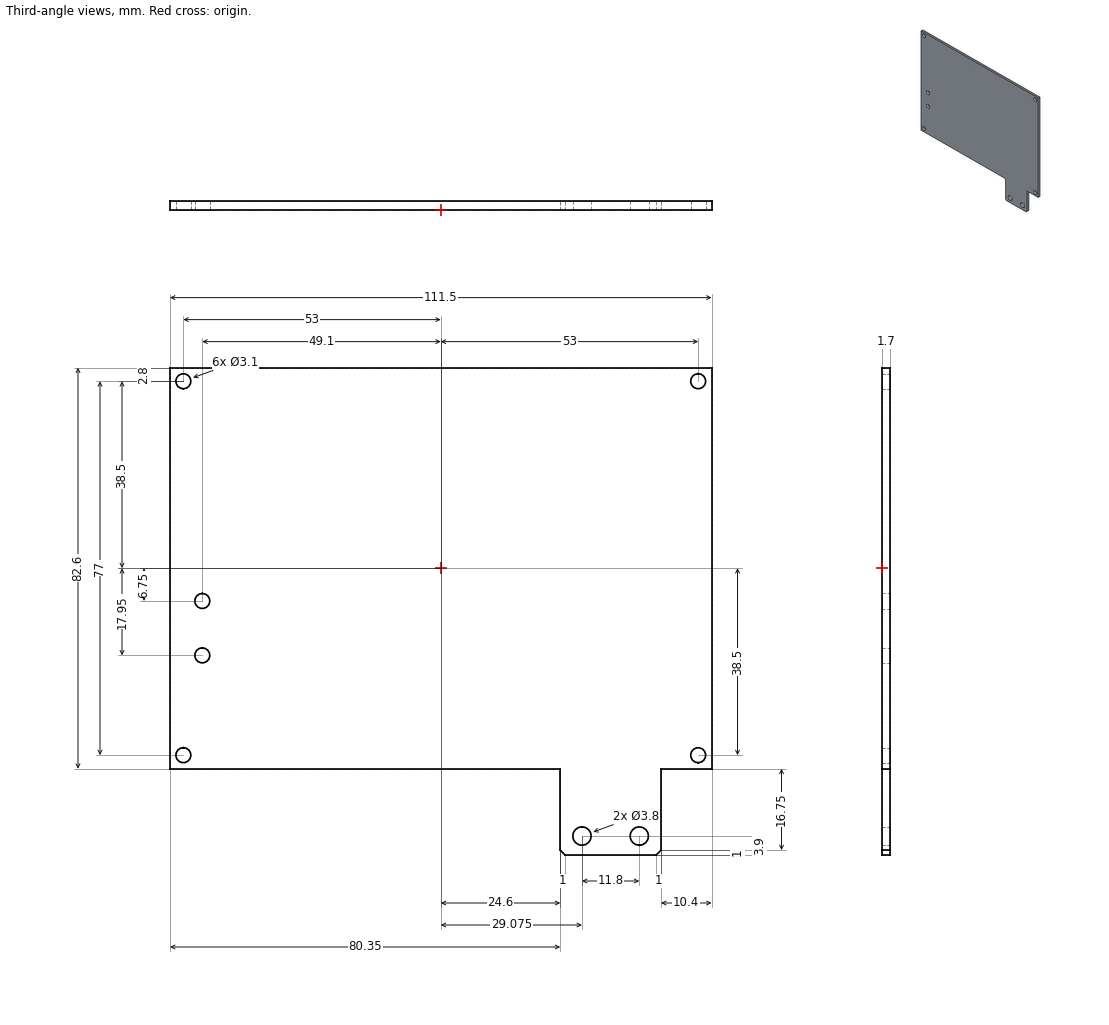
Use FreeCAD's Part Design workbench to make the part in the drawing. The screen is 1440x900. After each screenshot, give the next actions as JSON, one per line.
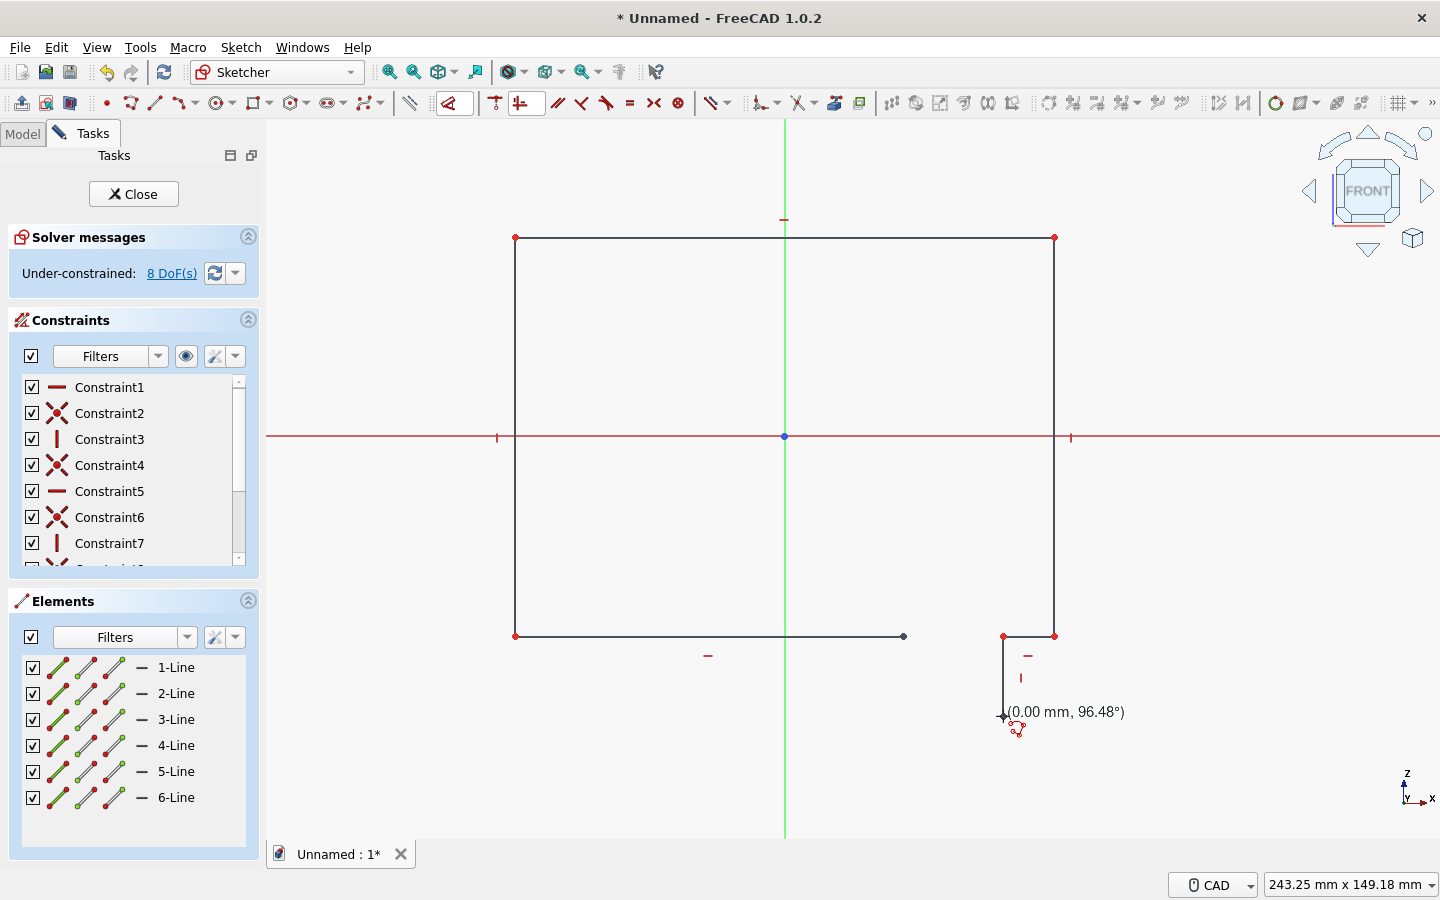
{"action": "scroll", "coordinate": [999, 721], "scroll_direction": "up", "scroll_amount": 5}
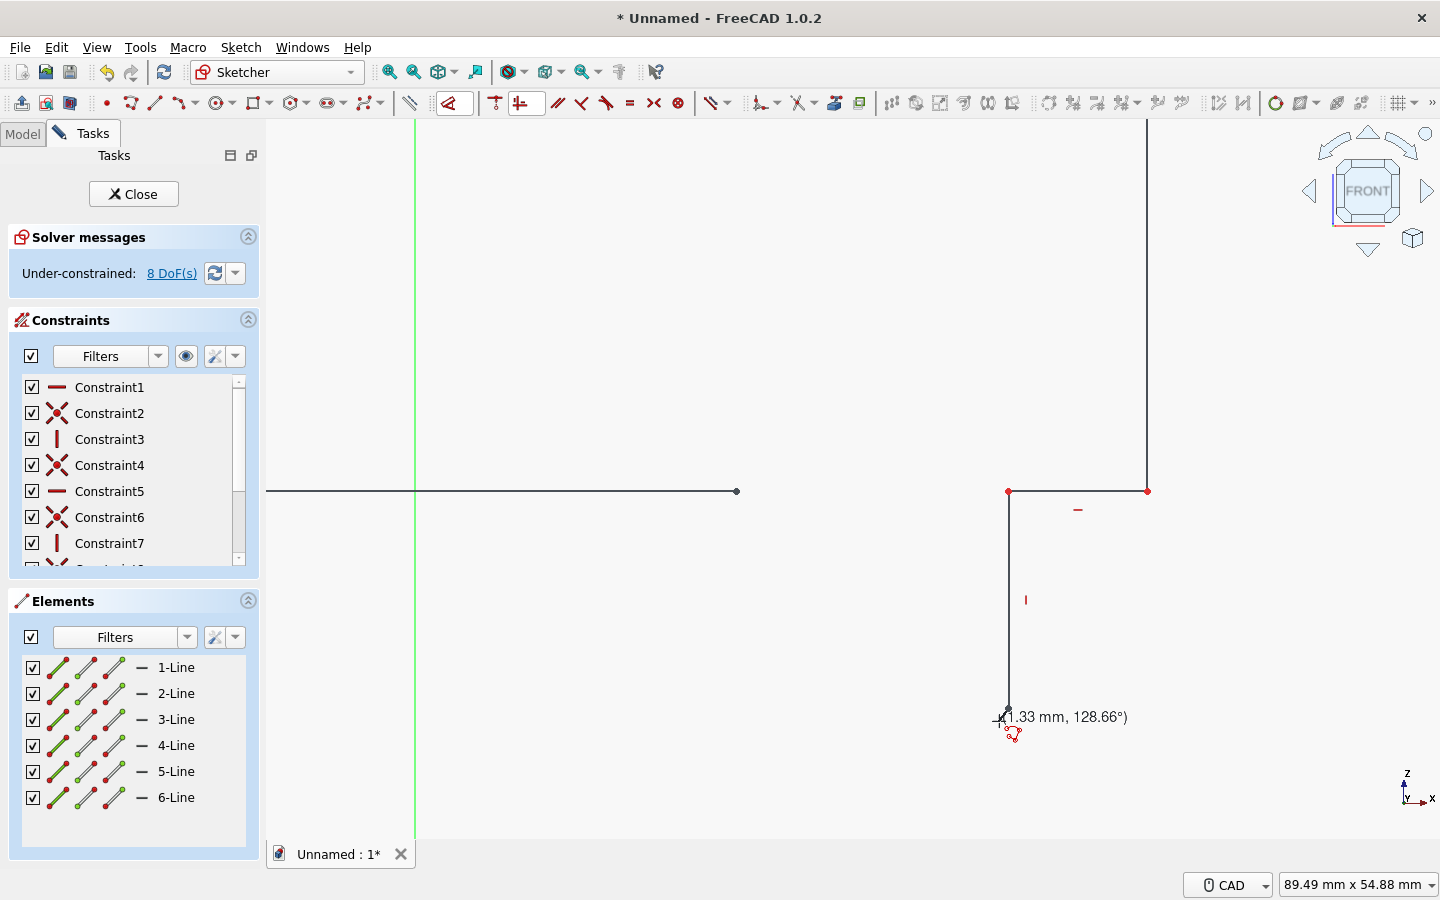
{"action": "left_click", "coordinate": [997, 720]}
{"action": "left_click", "coordinate": [751, 720]}
{"action": "left_click", "coordinate": [738, 707]}
{"action": "left_click", "coordinate": [737, 491]}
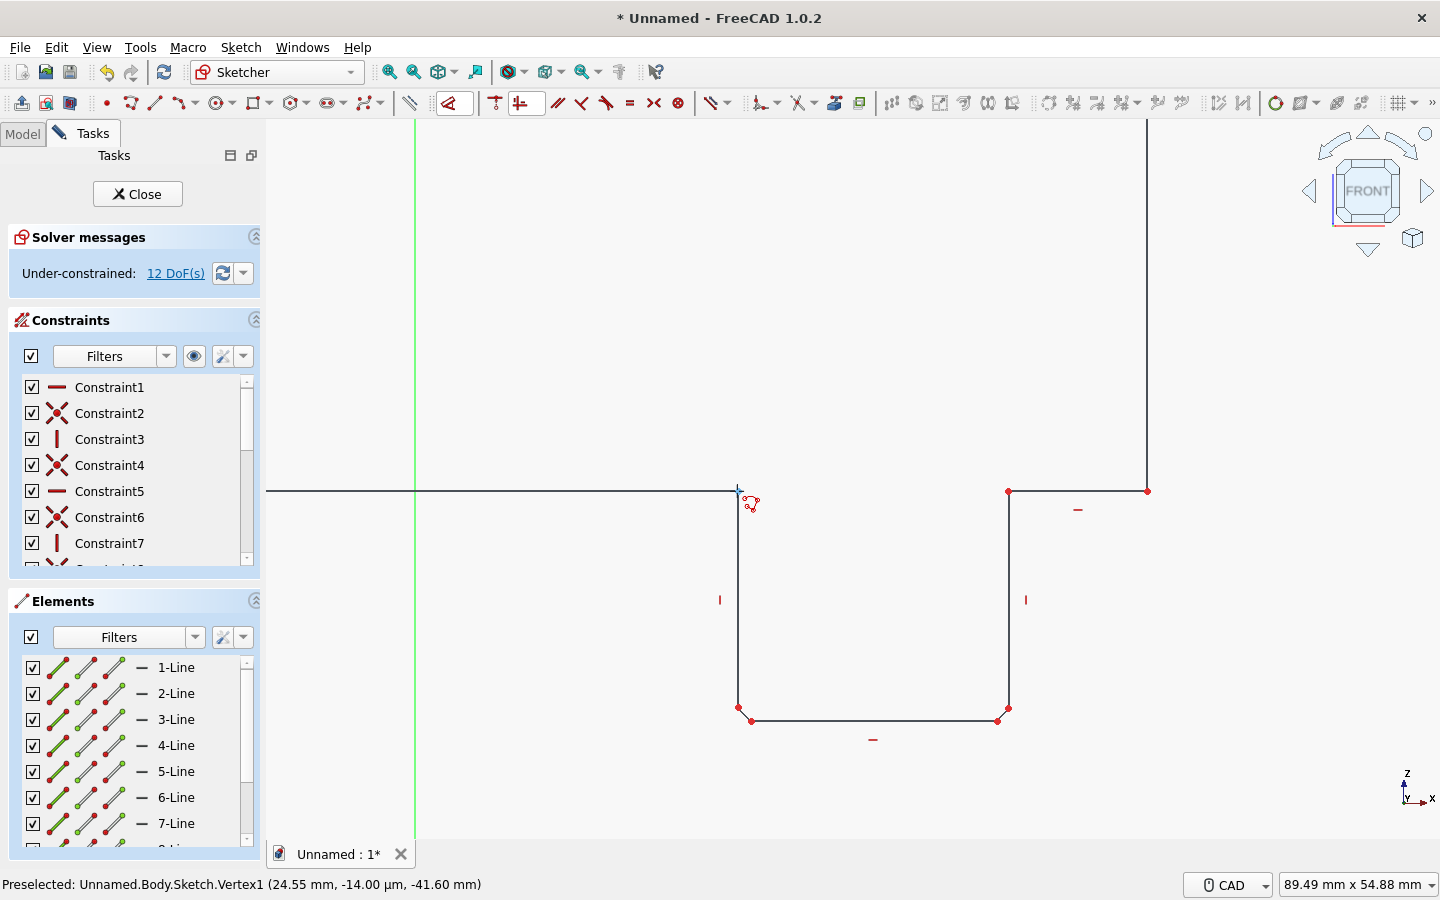
{"action": "left_click", "coordinate": [216, 104]}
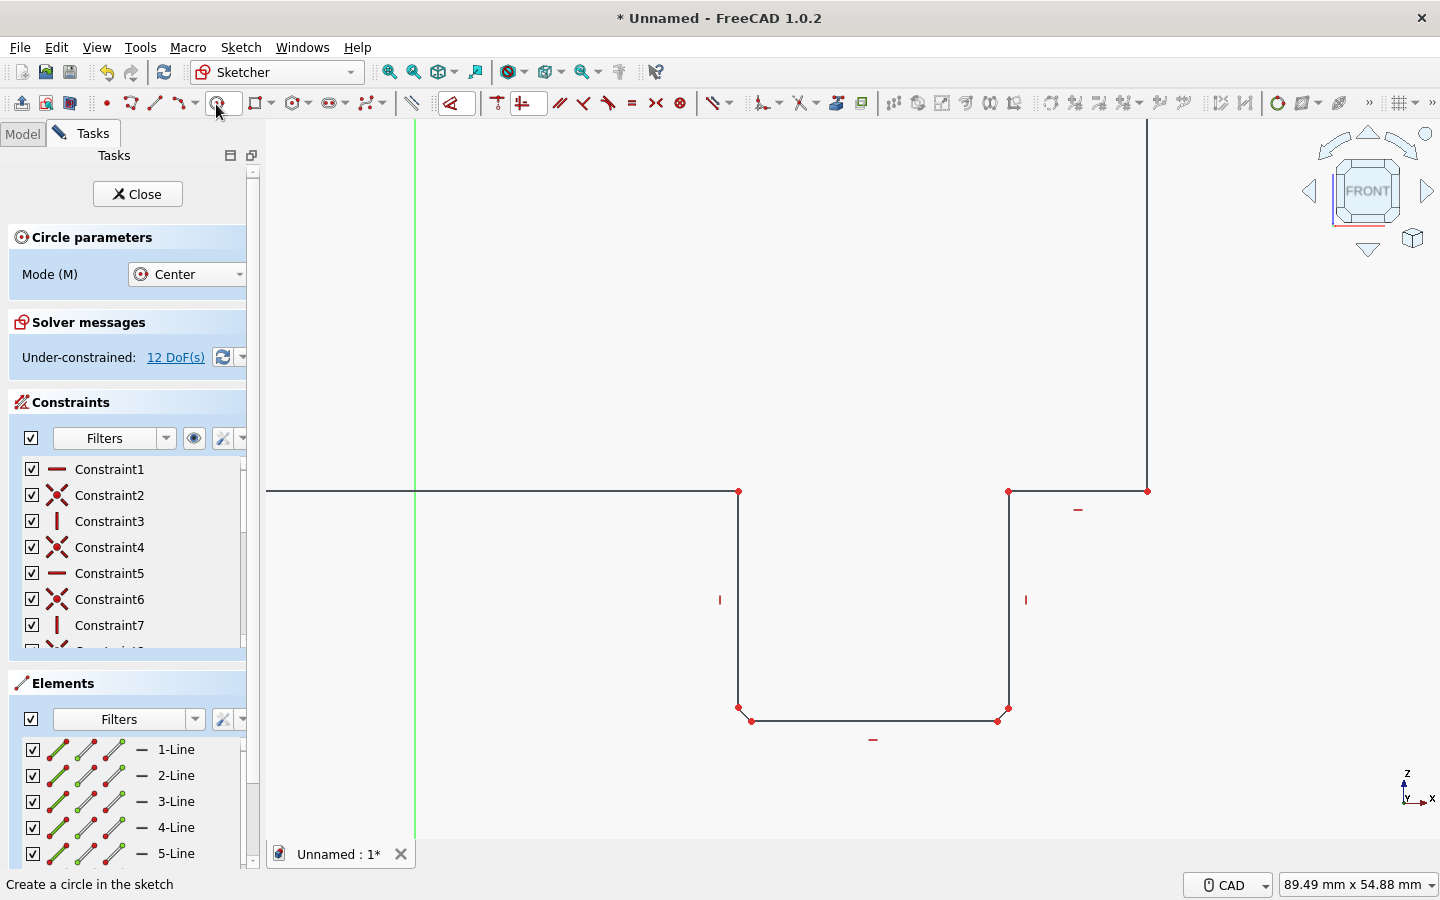
{"action": "scroll", "coordinate": [1000, 722], "scroll_direction": "down", "scroll_amount": 5}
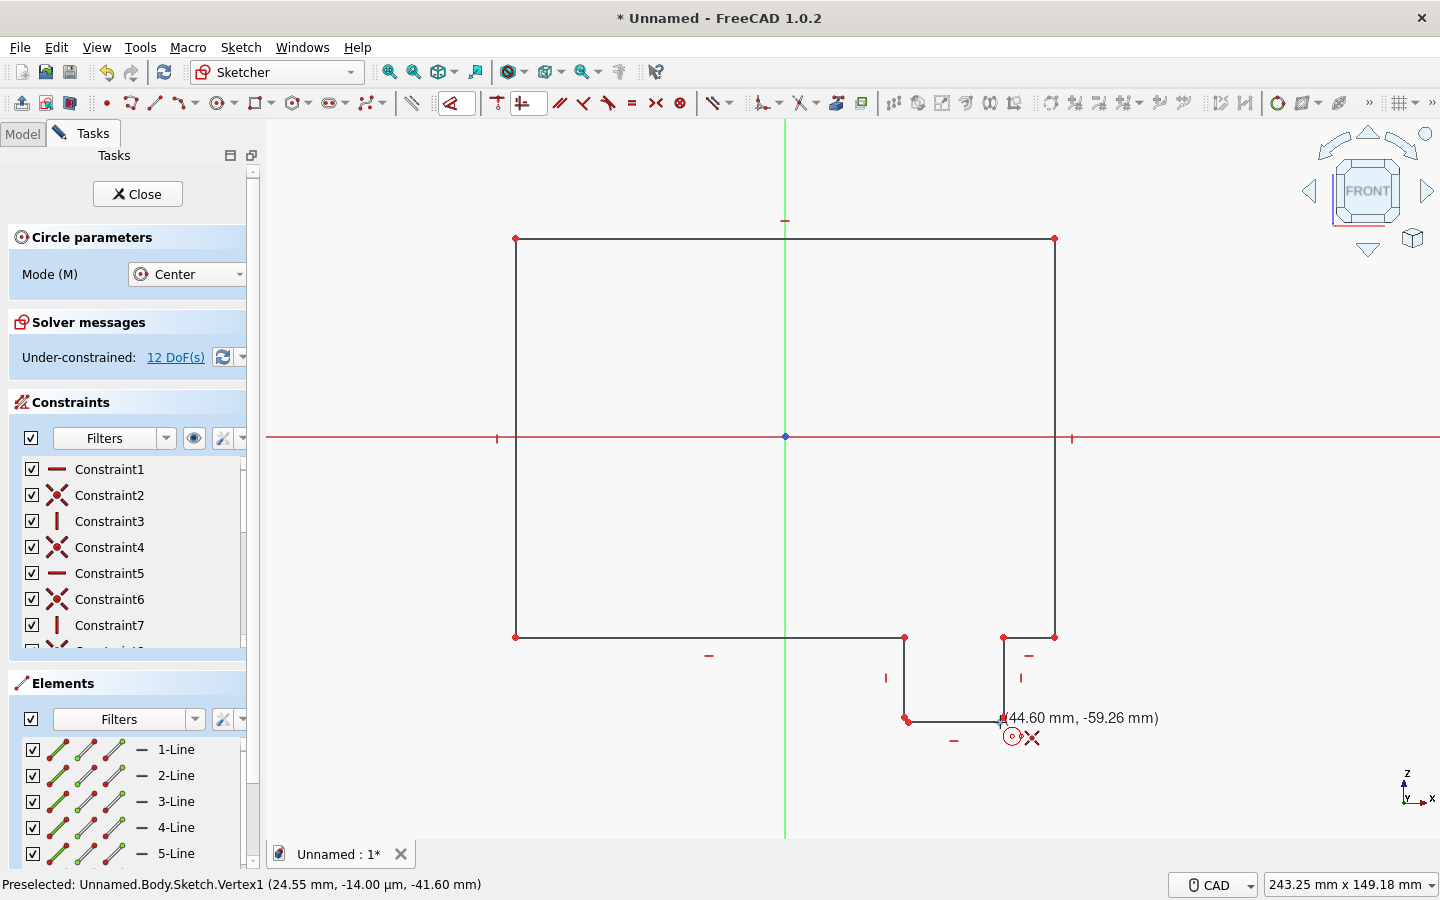
{"action": "scroll", "coordinate": [529, 251], "scroll_direction": "up", "scroll_amount": 6}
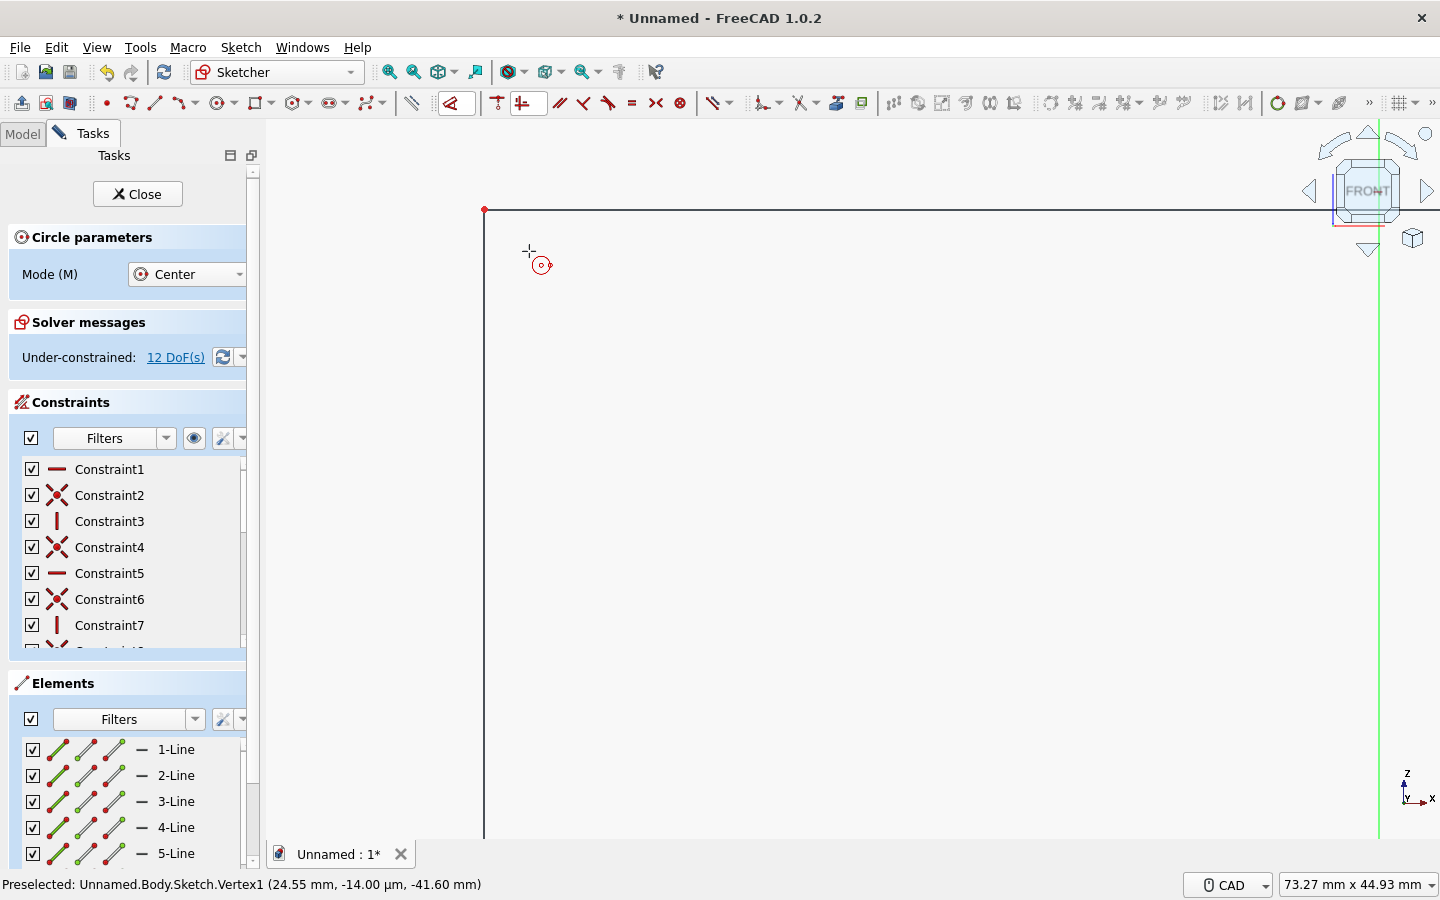
{"action": "left_click", "coordinate": [530, 251]}
{"action": "left_click", "coordinate": [547, 233]}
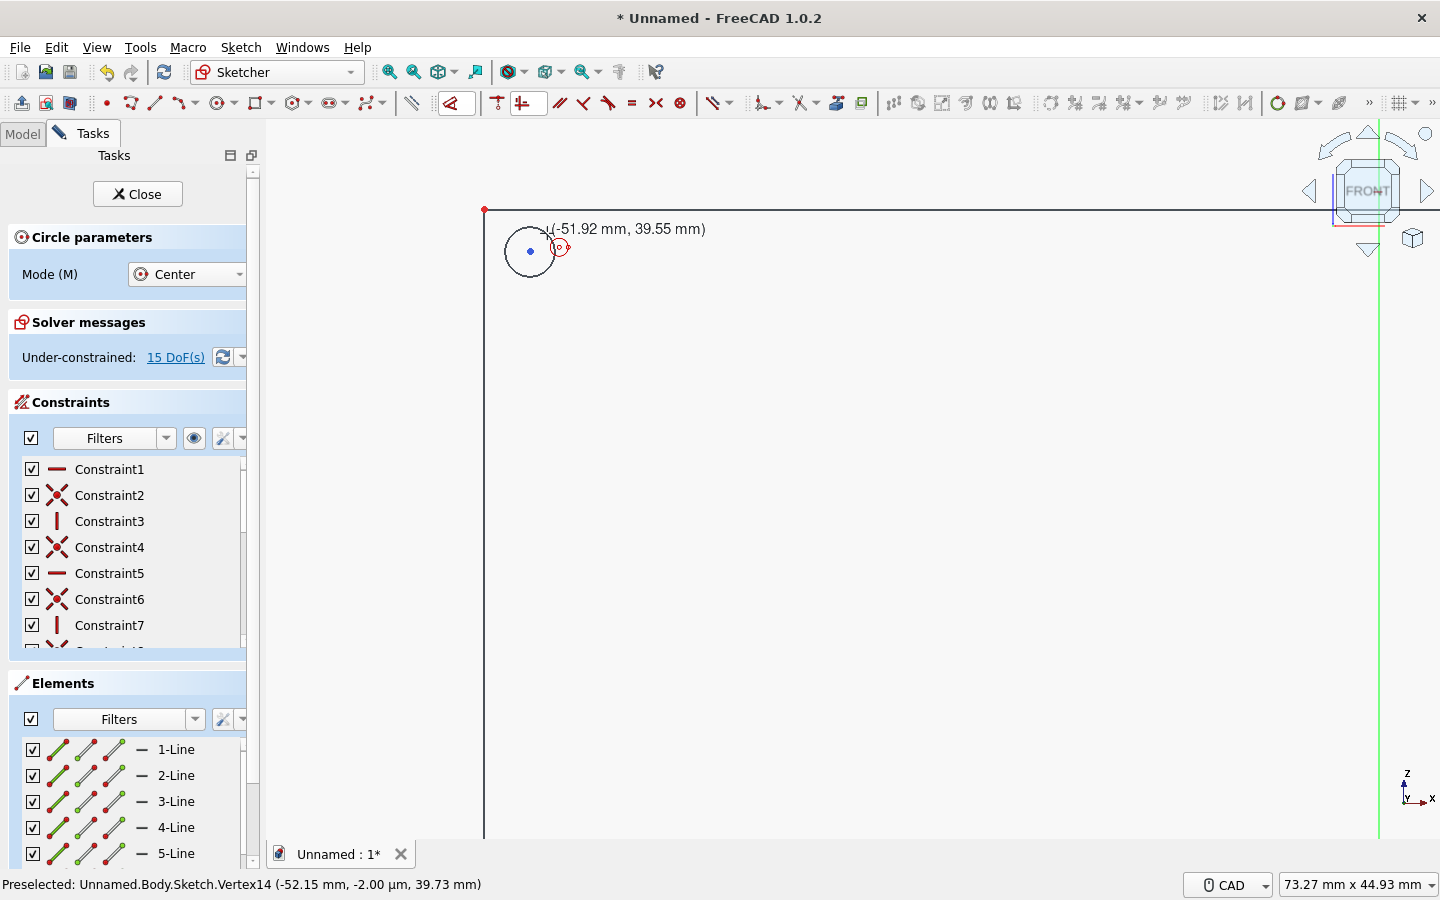
{"action": "scroll", "coordinate": [528, 250], "scroll_direction": "down", "scroll_amount": 6}